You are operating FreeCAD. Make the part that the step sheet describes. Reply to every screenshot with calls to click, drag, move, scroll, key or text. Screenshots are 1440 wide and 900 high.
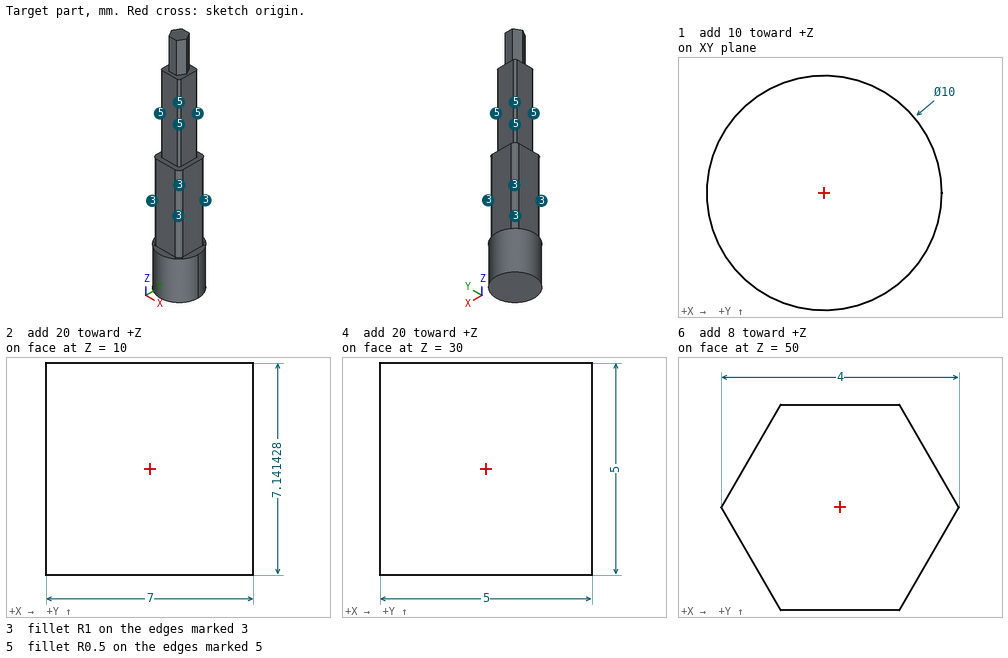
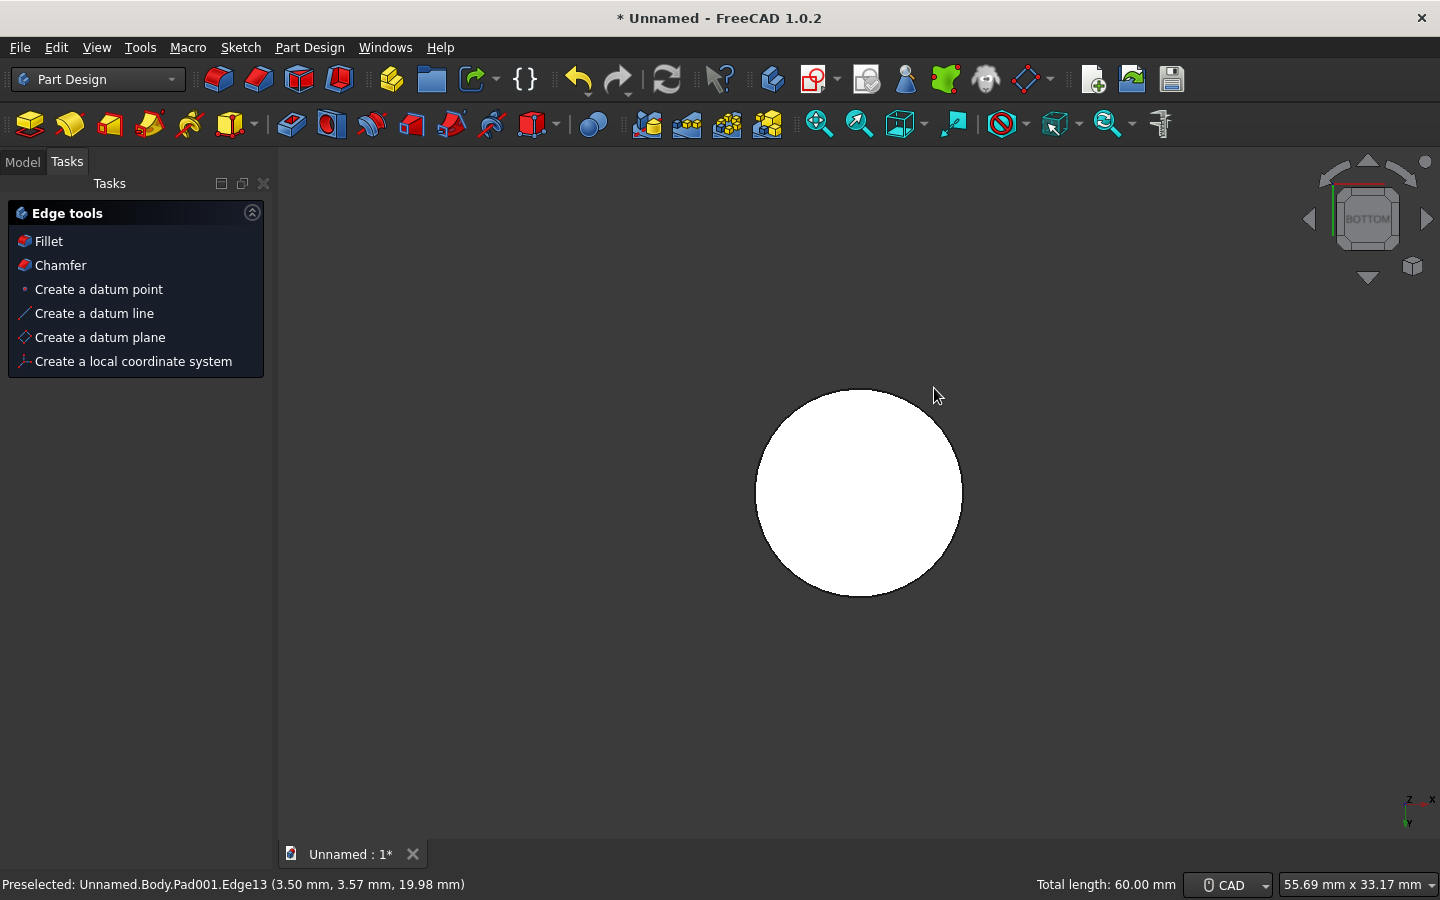
key(4)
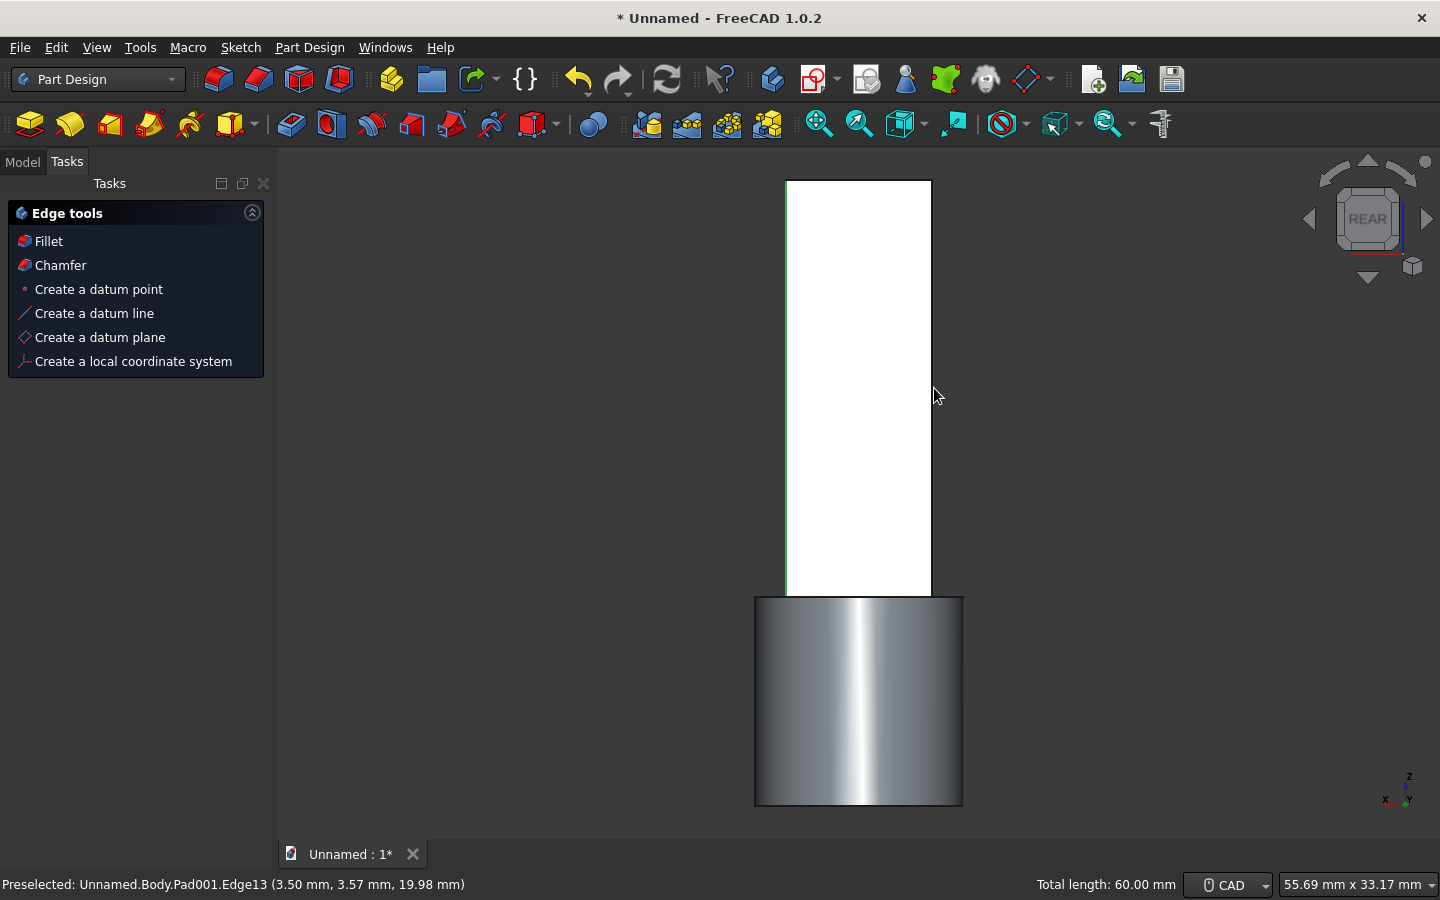
click(932, 388, ctrl)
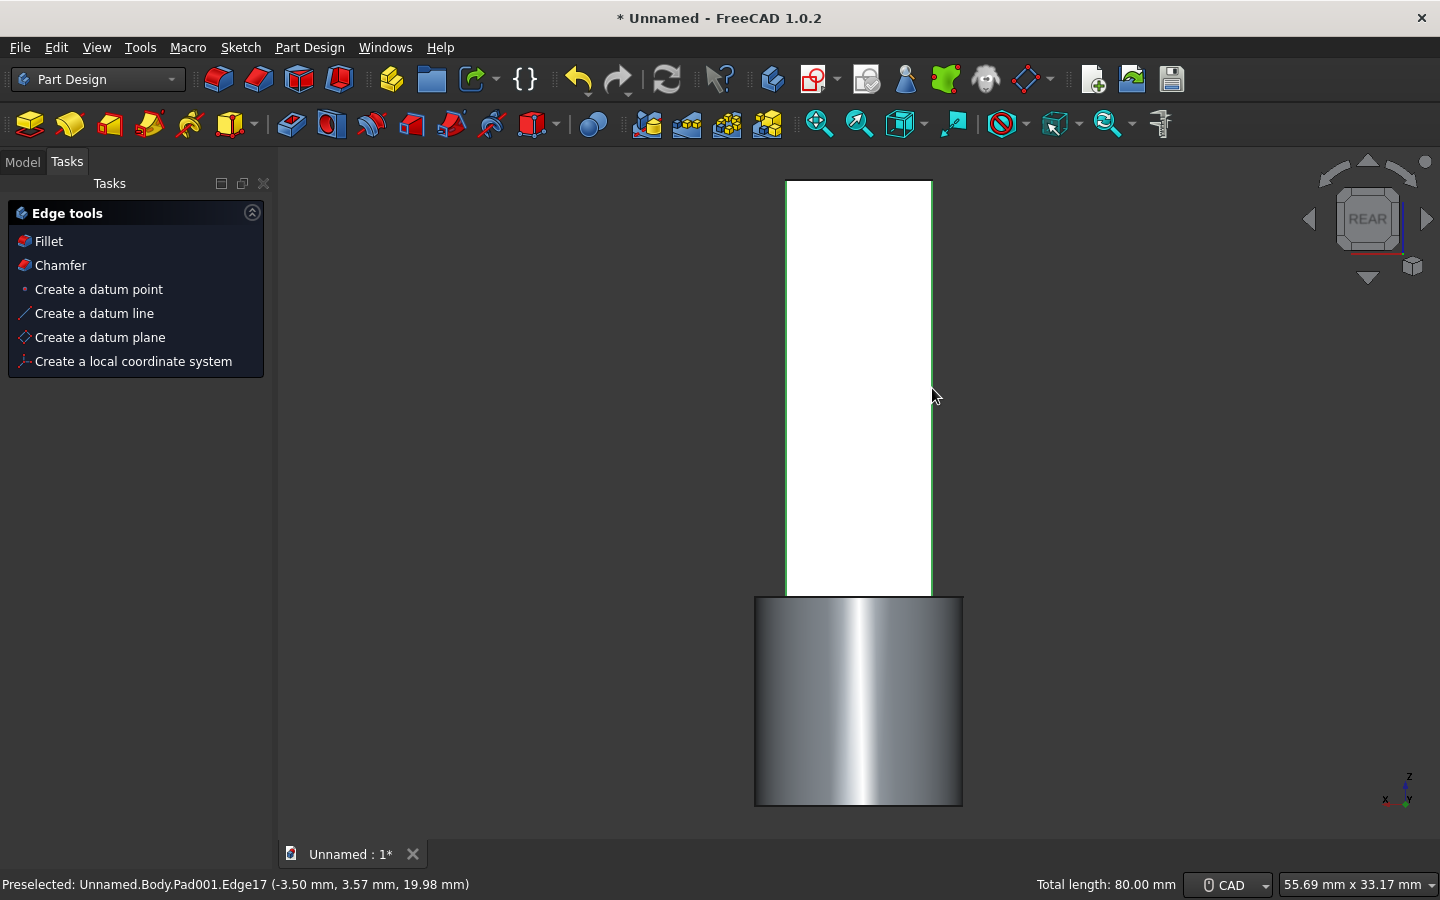
click(220, 80)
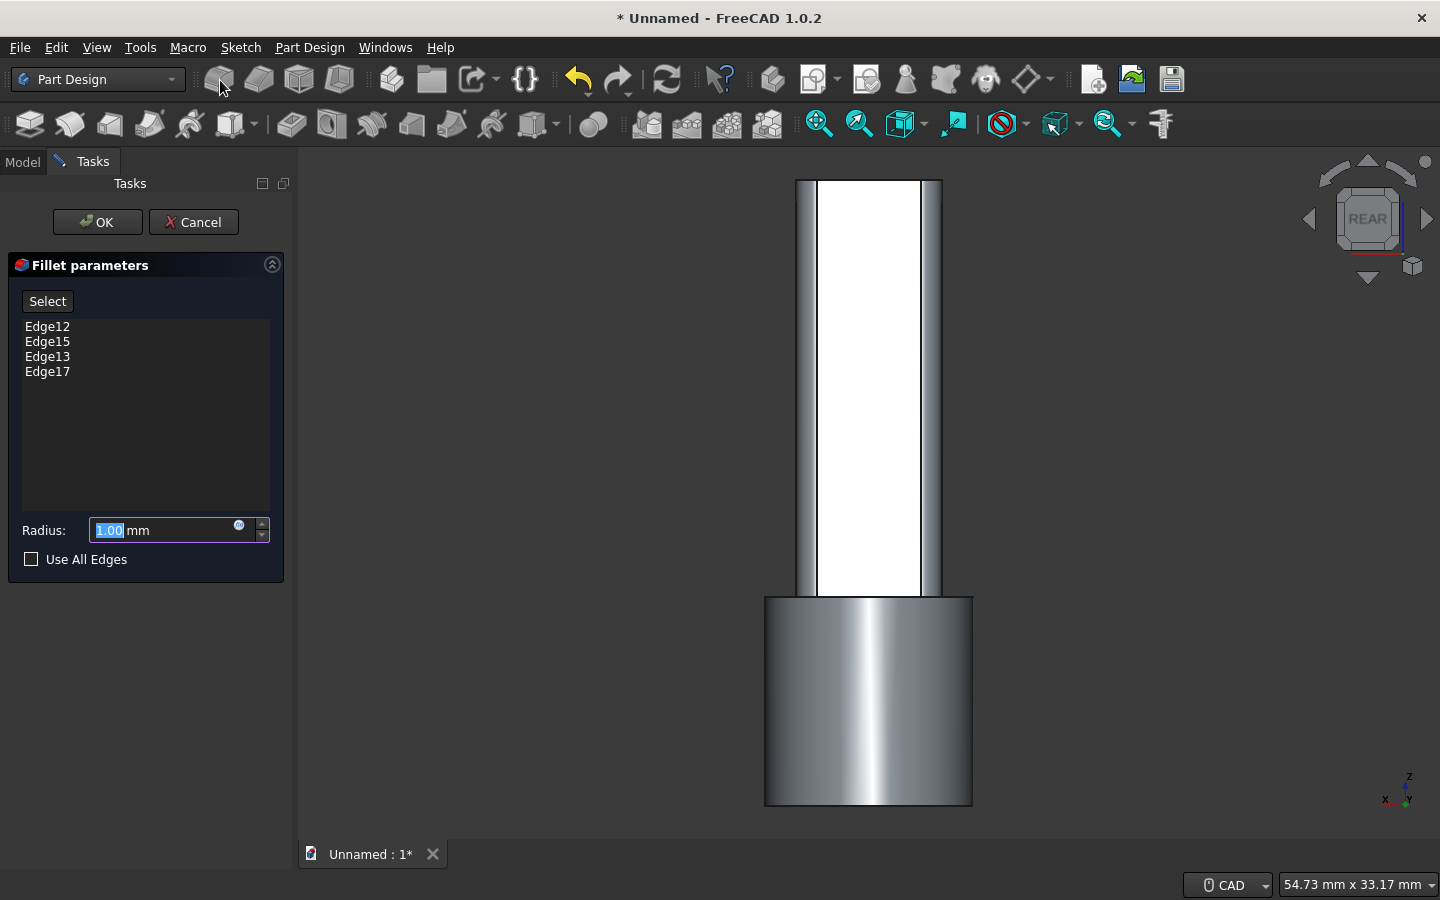
text(1)
key(Tab)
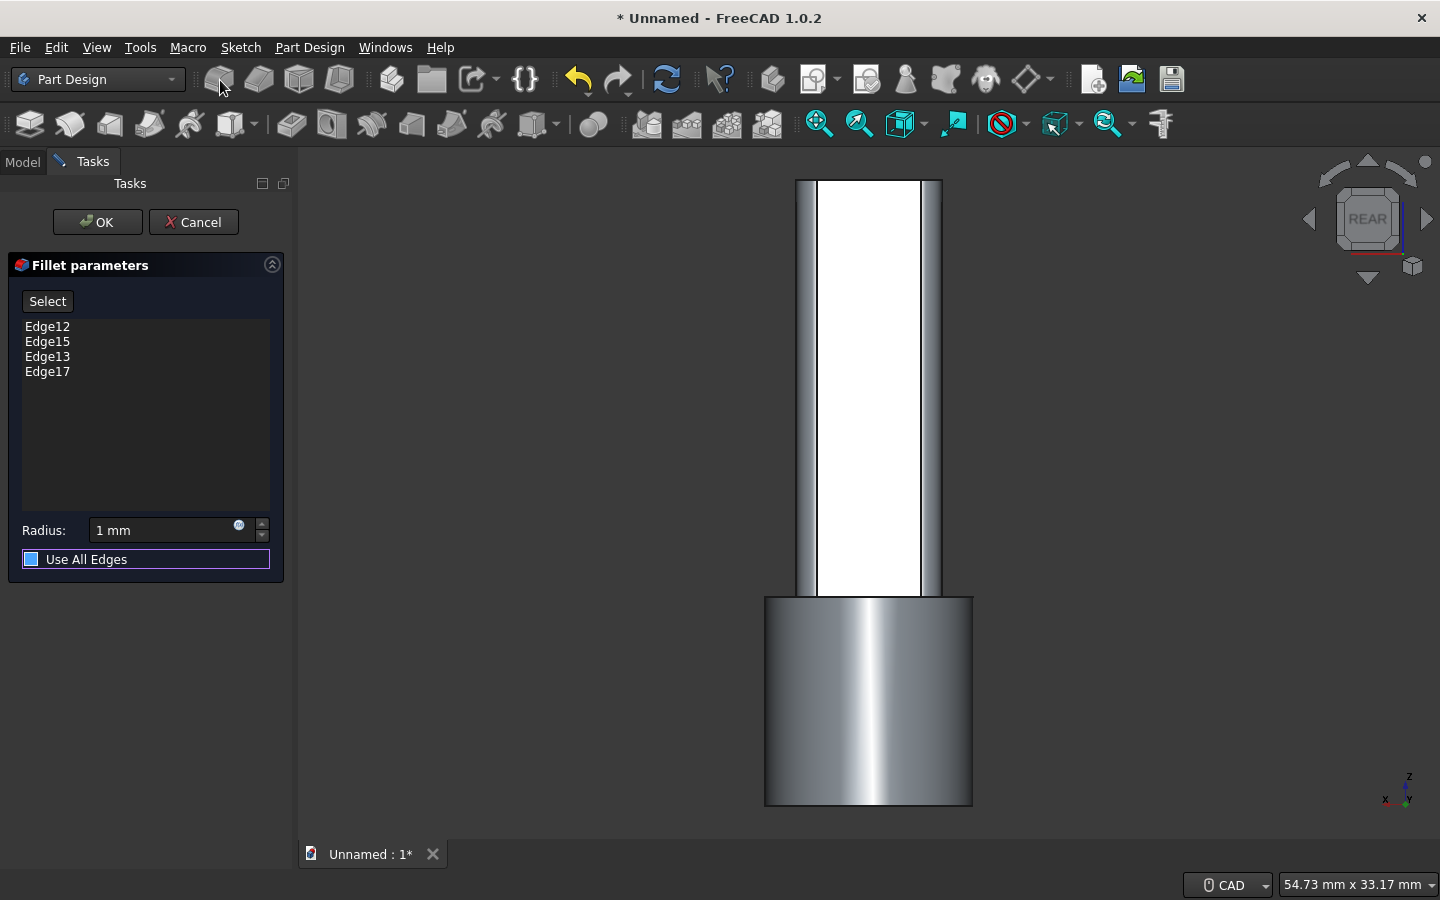
click(98, 222)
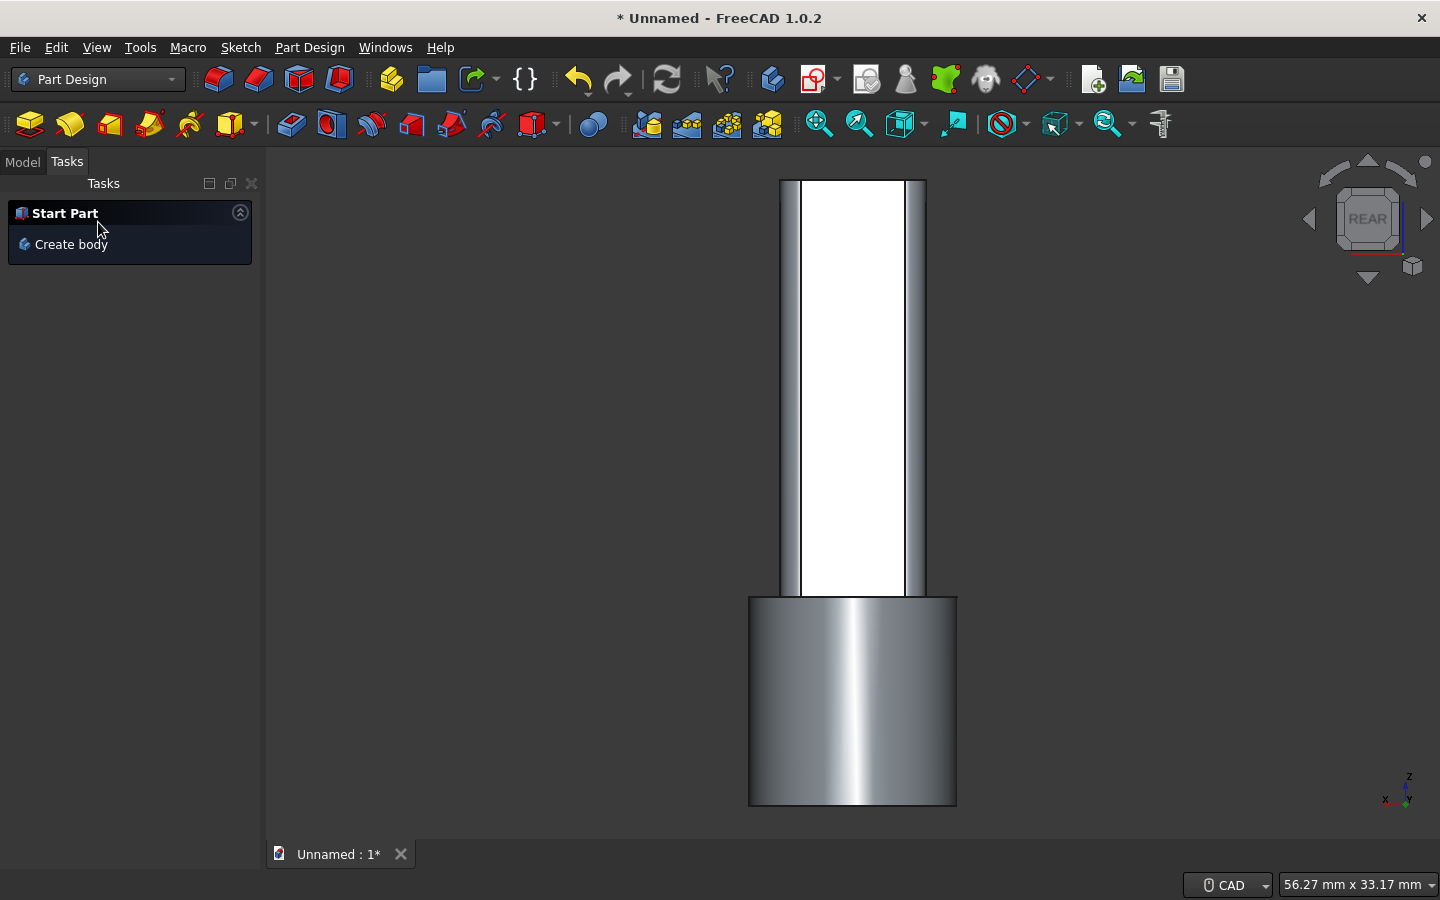
key(0)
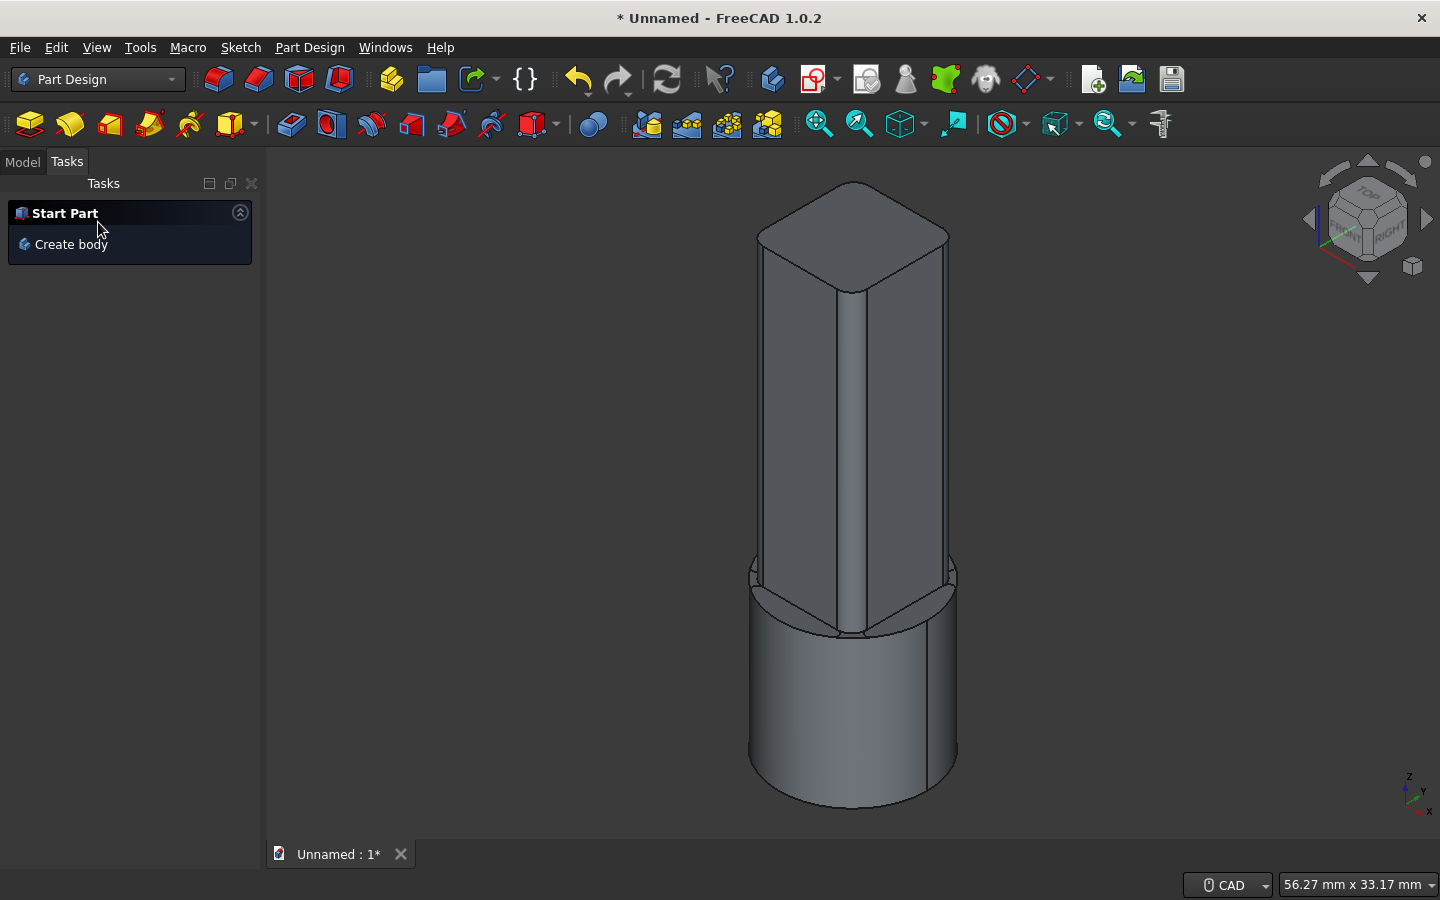
click(853, 236)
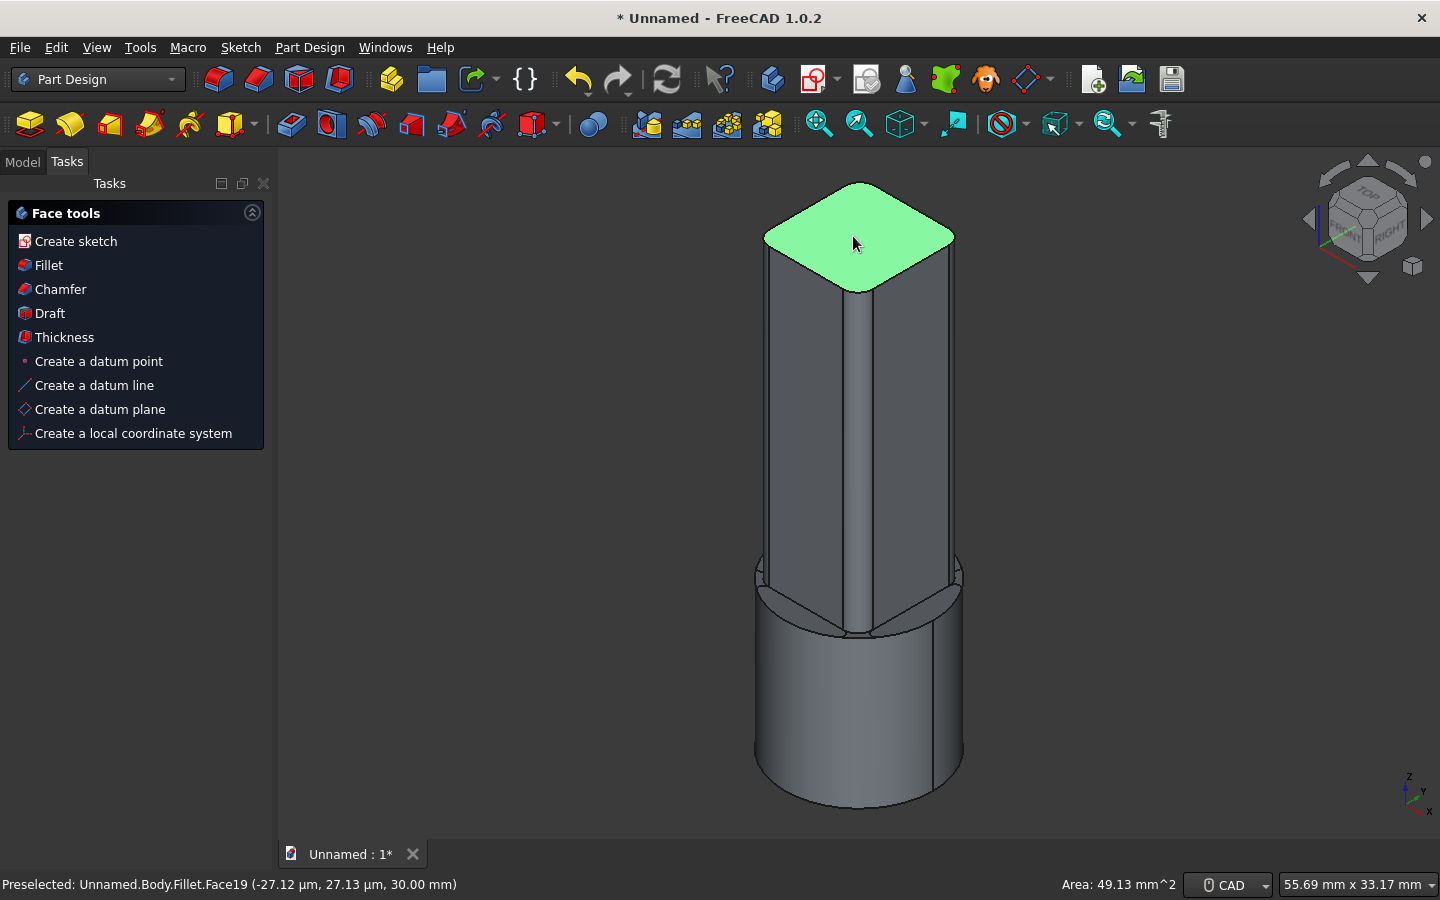
click(814, 80)